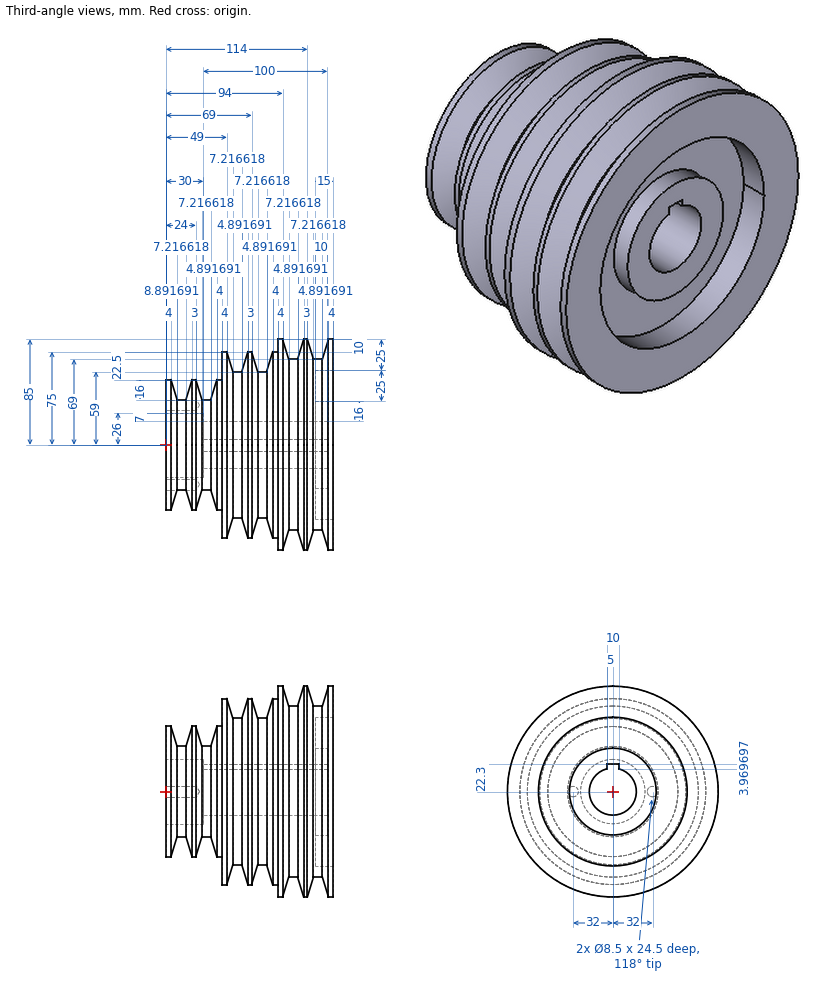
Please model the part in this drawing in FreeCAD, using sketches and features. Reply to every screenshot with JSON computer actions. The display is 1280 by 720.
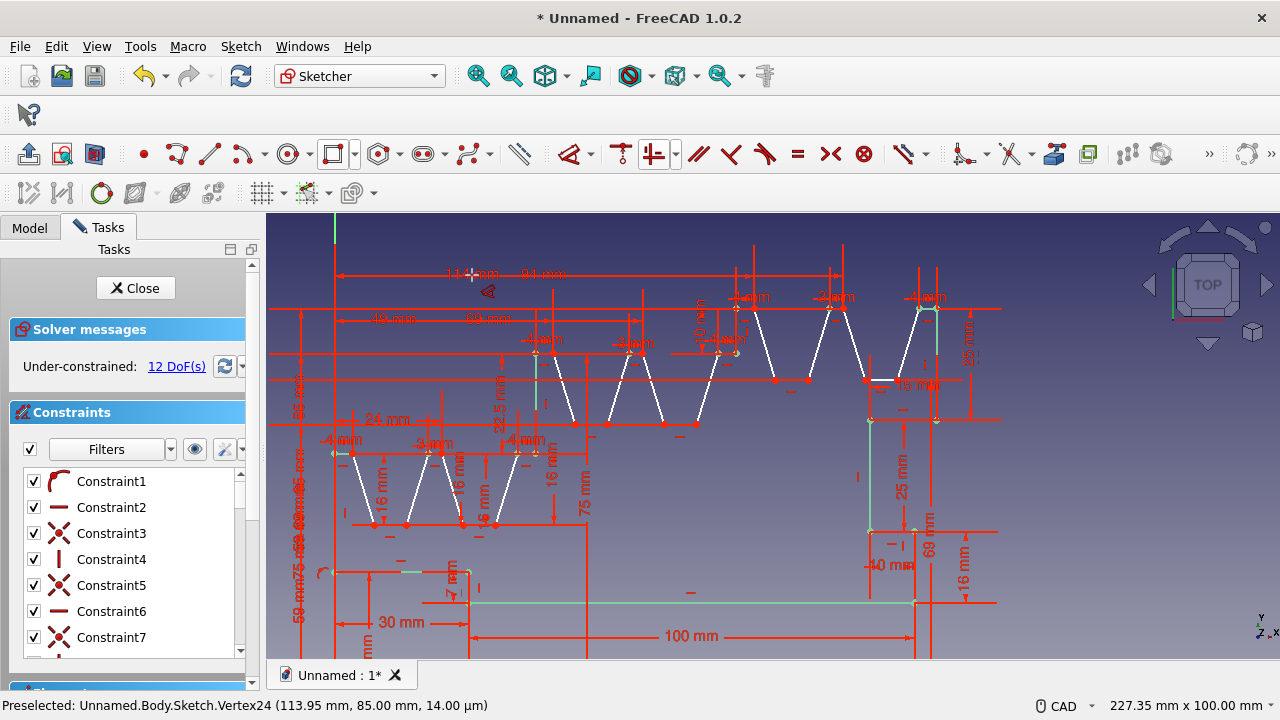
{"action": "scroll", "coordinate": [888, 380], "scroll_direction": "up", "scroll_amount": 2}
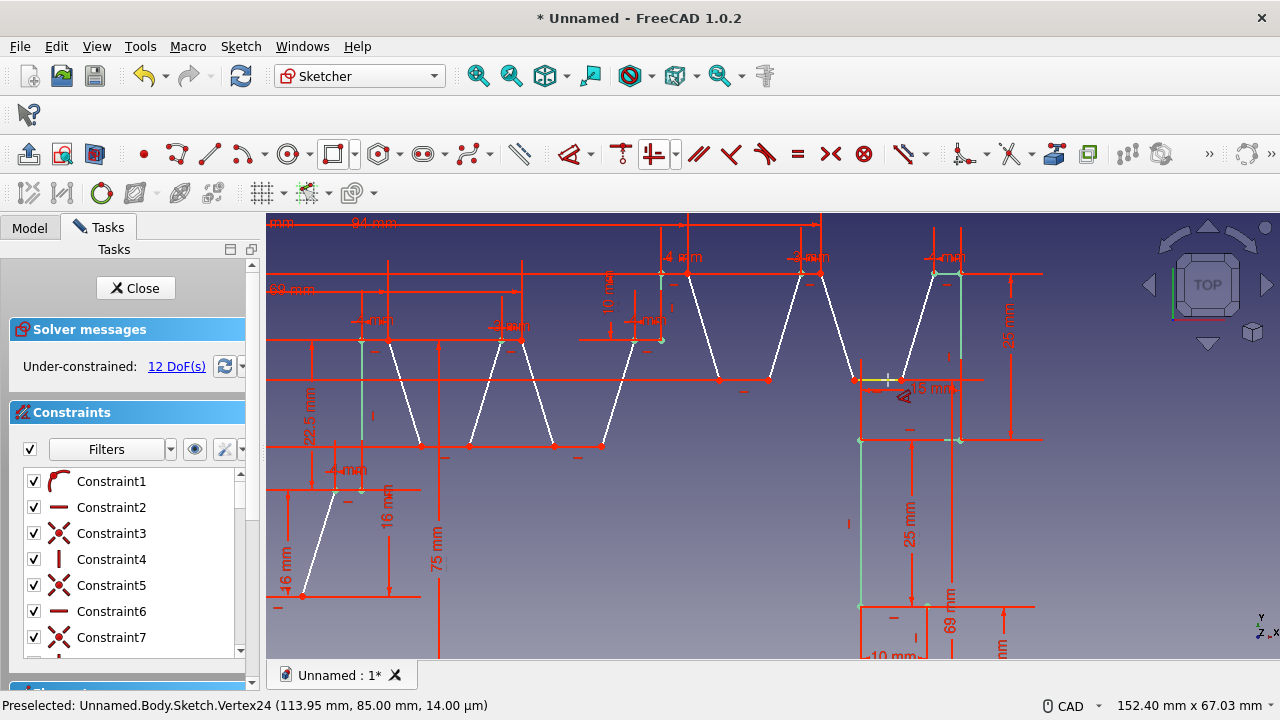
{"action": "left_click", "coordinate": [887, 380]}
{"action": "left_click", "coordinate": [878, 346]}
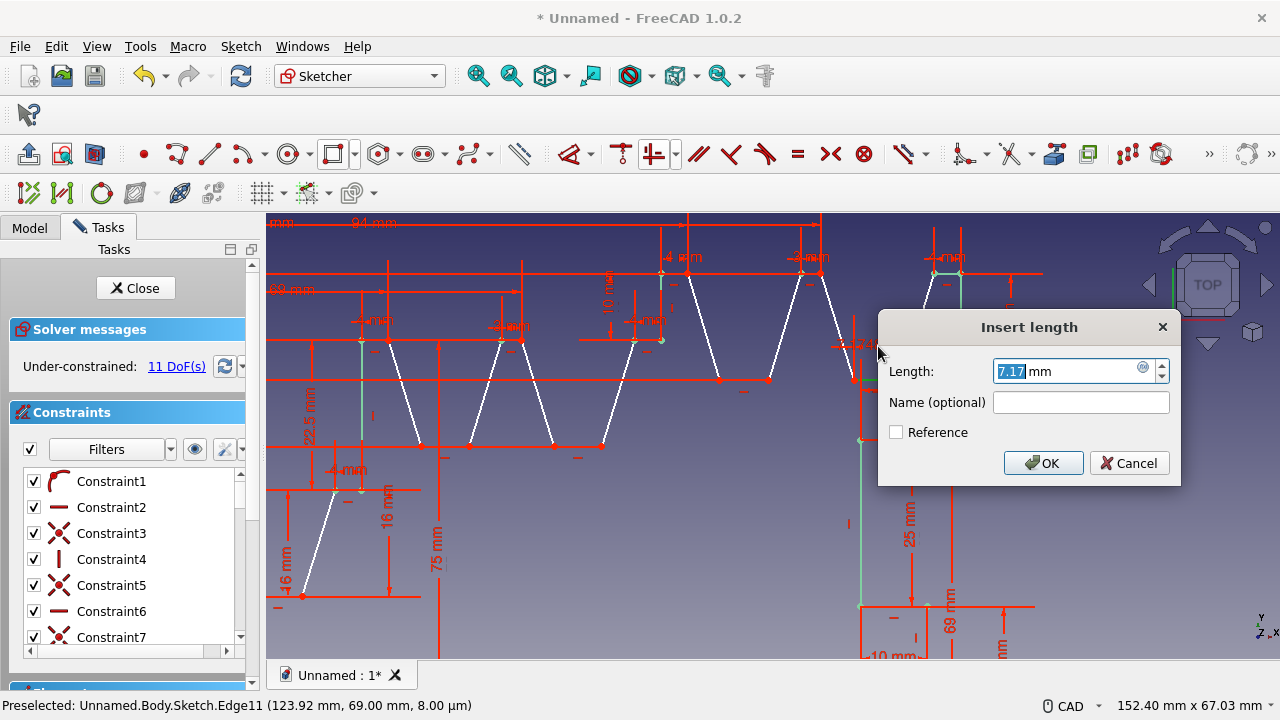
{"action": "type", "text": "7.216618"}
{"action": "key", "text": "Return"}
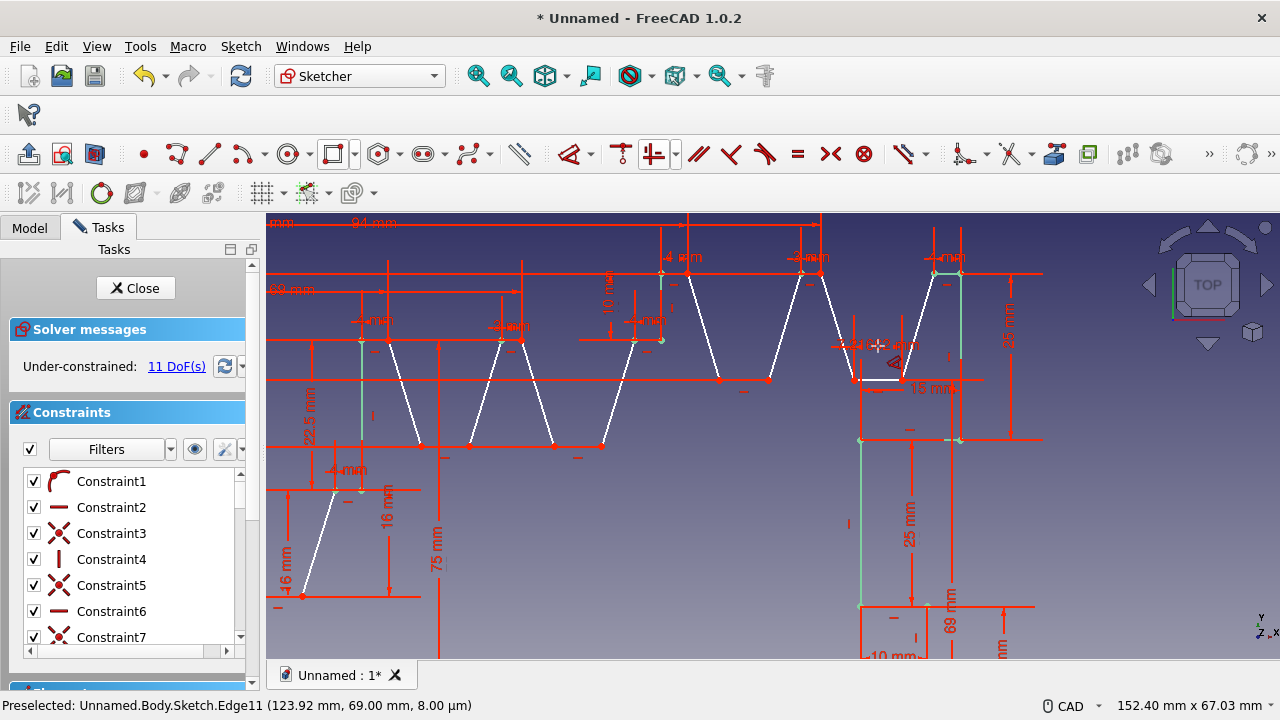
{"action": "left_click", "coordinate": [754, 380]}
{"action": "left_click", "coordinate": [744, 346]}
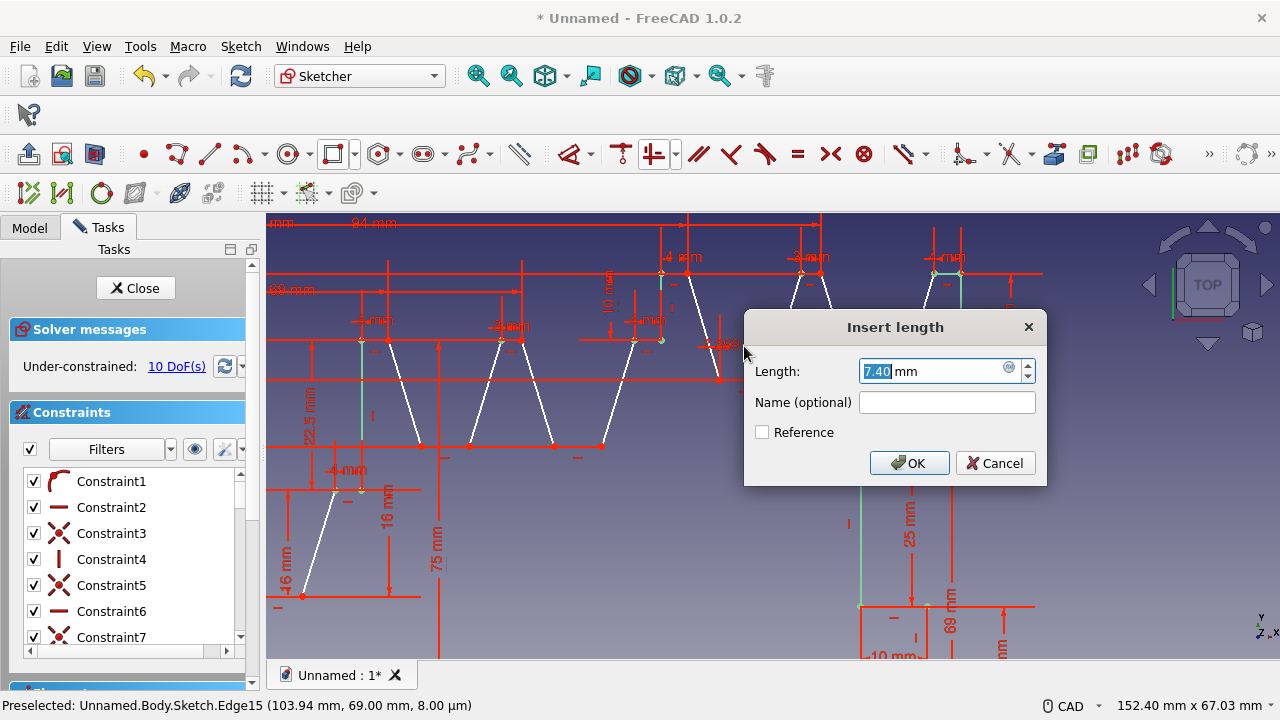
{"action": "type", "text": "7.216618"}
{"action": "key", "text": "Return"}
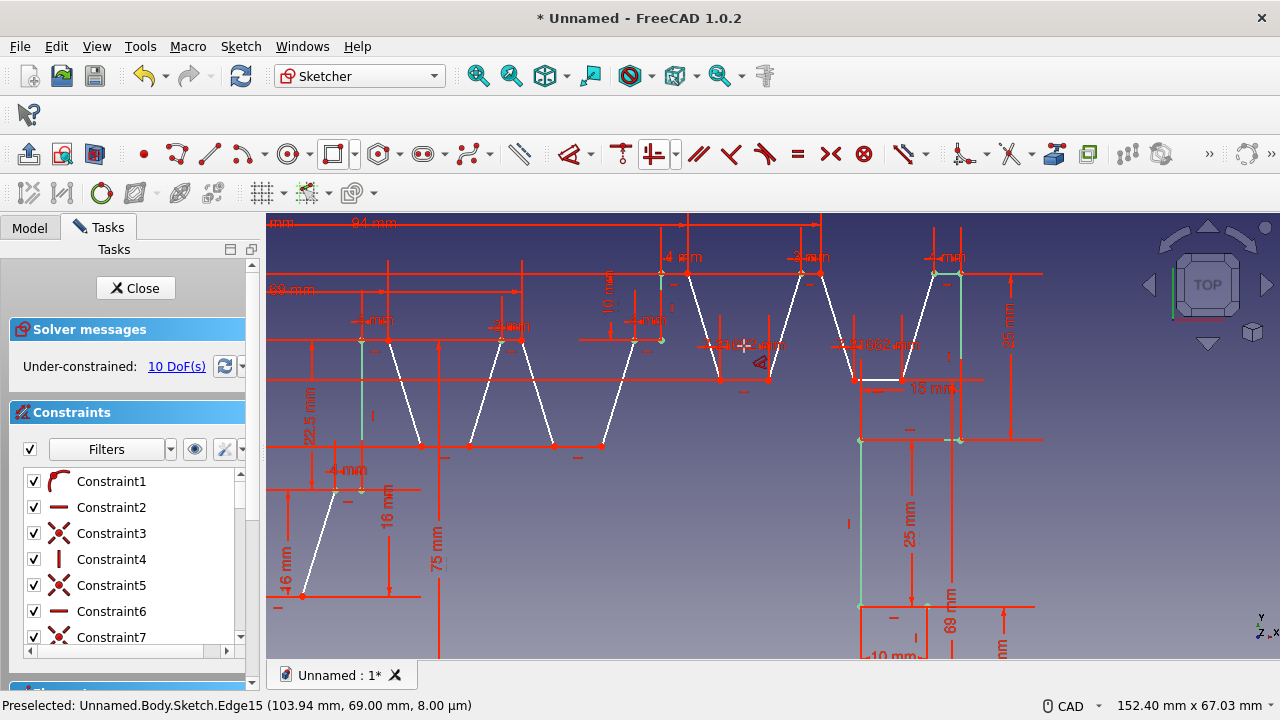
{"action": "left_click", "coordinate": [588, 447]}
{"action": "left_click", "coordinate": [578, 413]}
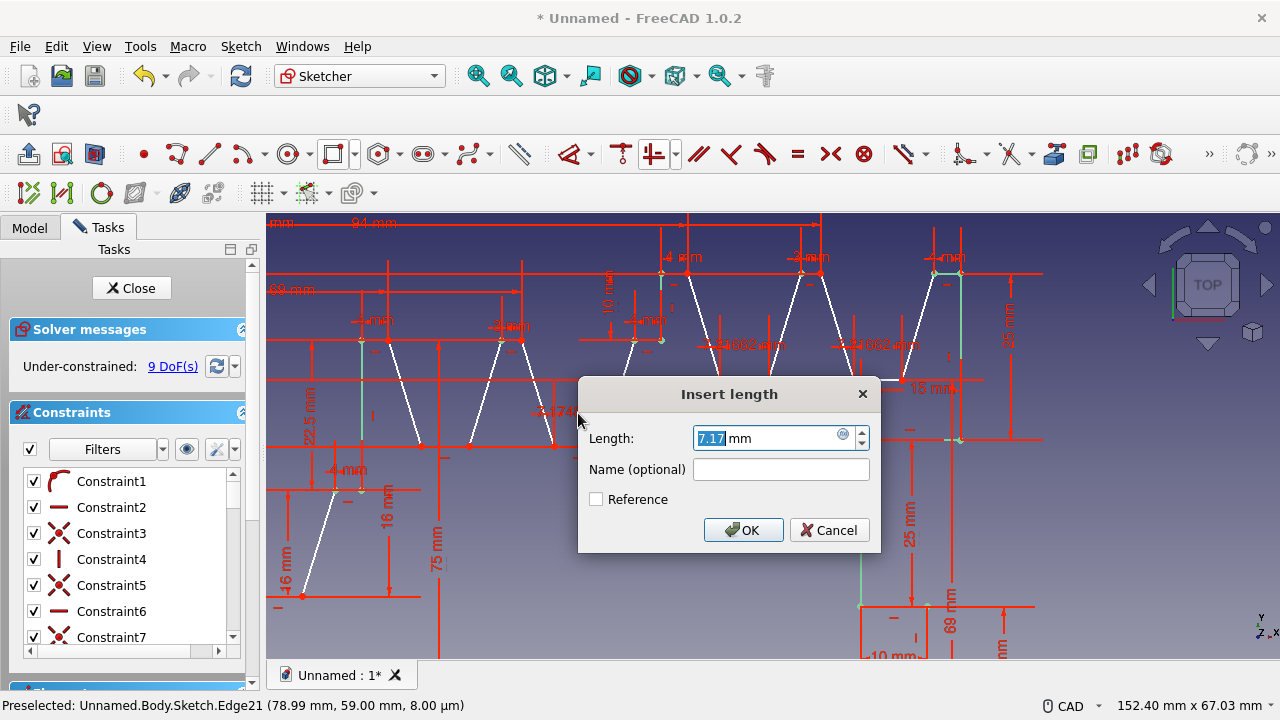
{"action": "type", "text": "7.216618"}
{"action": "key", "text": "Return"}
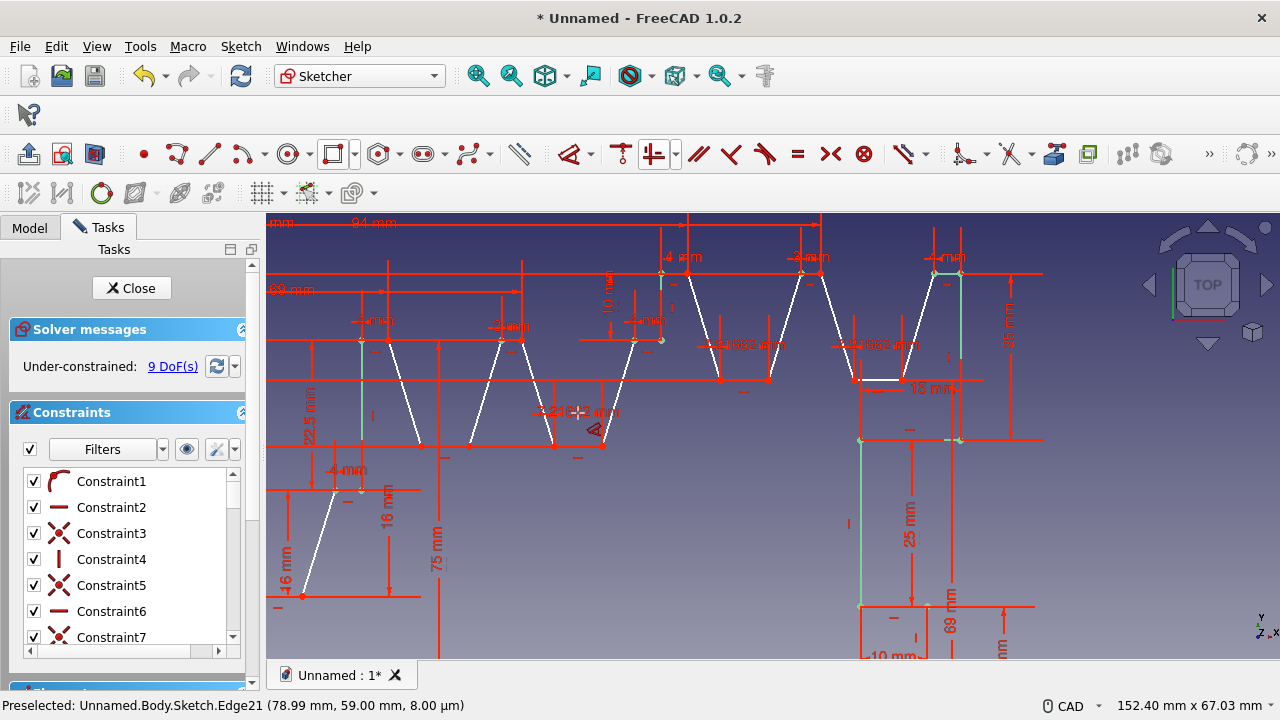
{"action": "left_click", "coordinate": [455, 447]}
{"action": "left_click", "coordinate": [445, 413]}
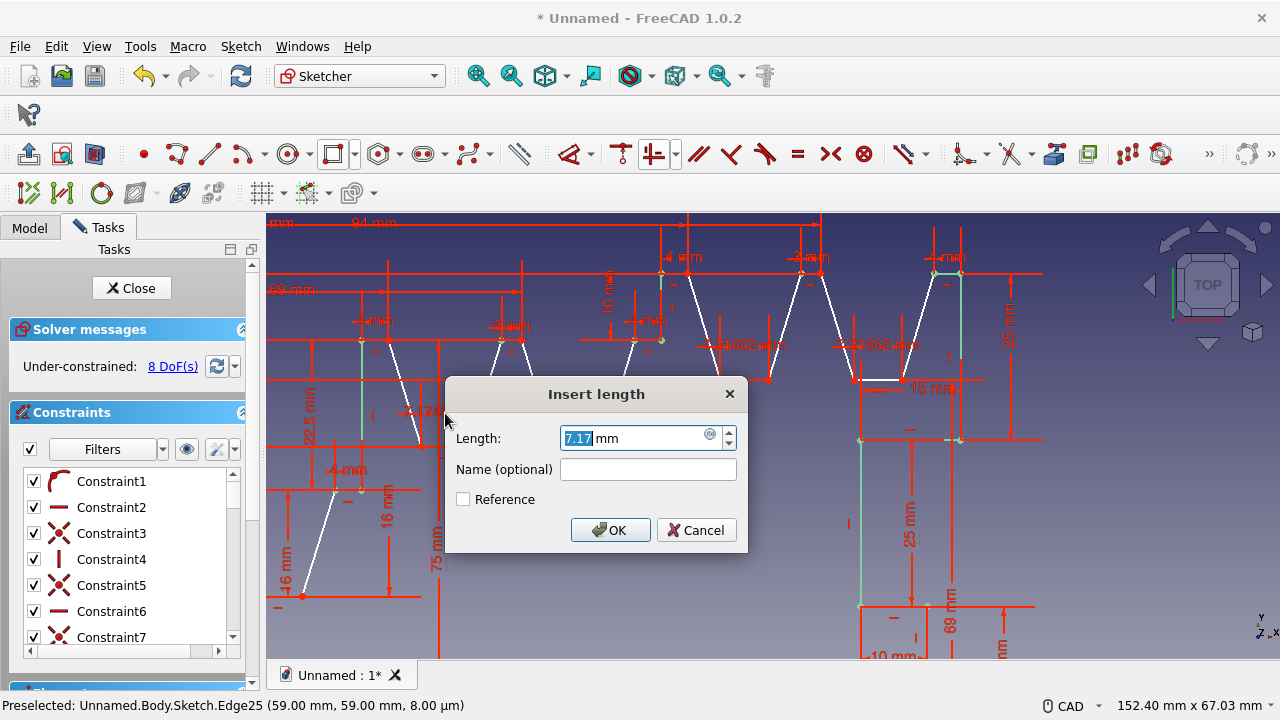
{"action": "type", "text": "7.216618"}
{"action": "key", "text": "Return"}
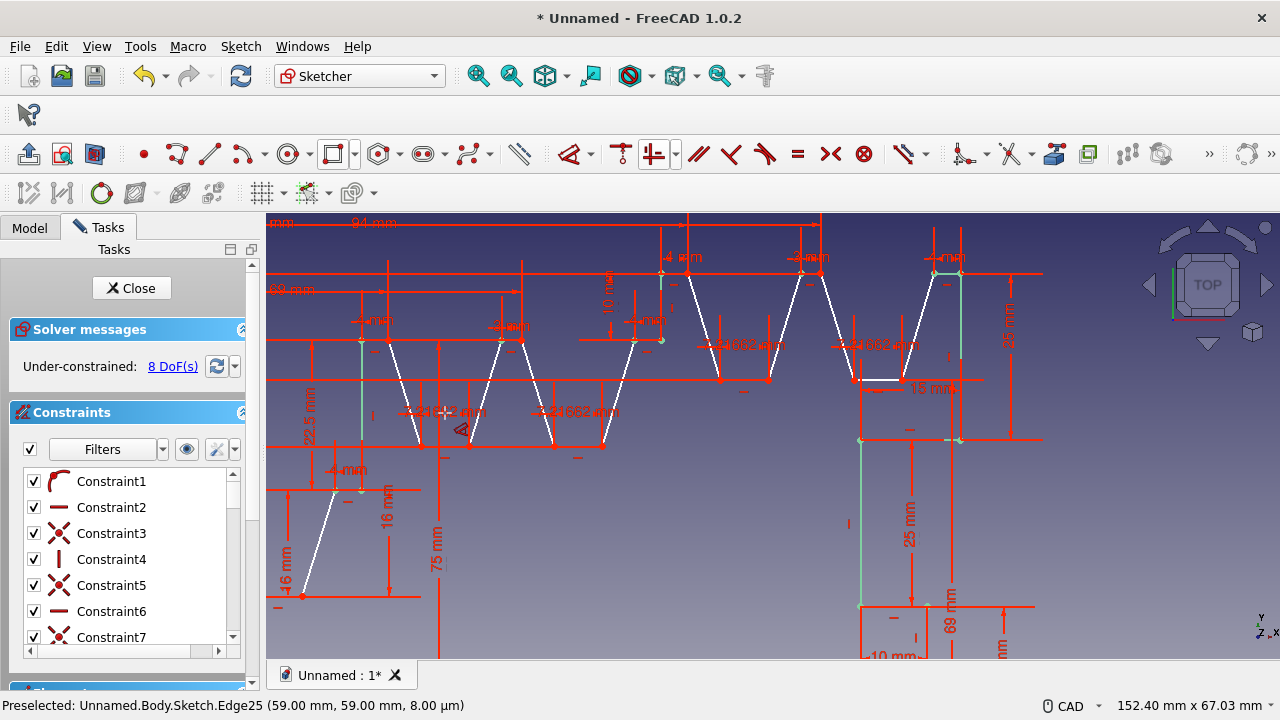
{"action": "scroll", "coordinate": [862, 338], "scroll_direction": "down", "scroll_amount": 4}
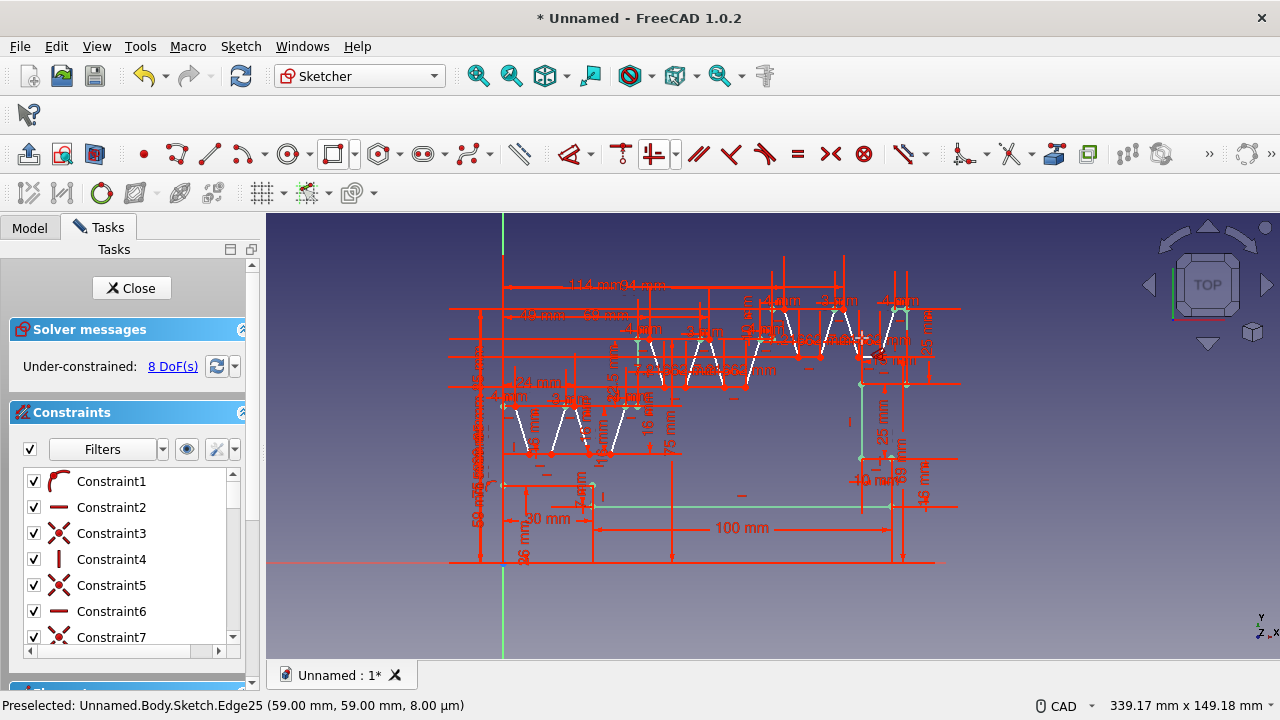
{"action": "scroll", "coordinate": [604, 454], "scroll_direction": "up", "scroll_amount": 4}